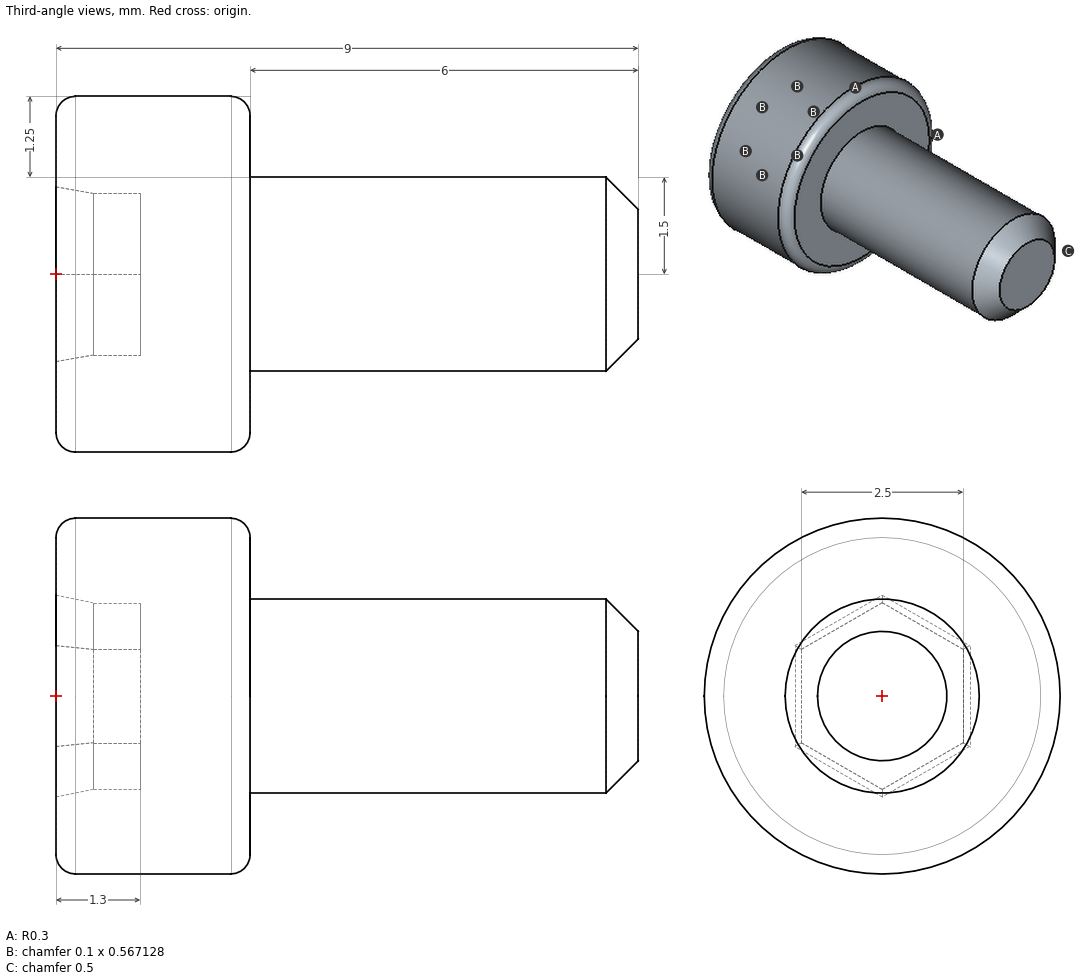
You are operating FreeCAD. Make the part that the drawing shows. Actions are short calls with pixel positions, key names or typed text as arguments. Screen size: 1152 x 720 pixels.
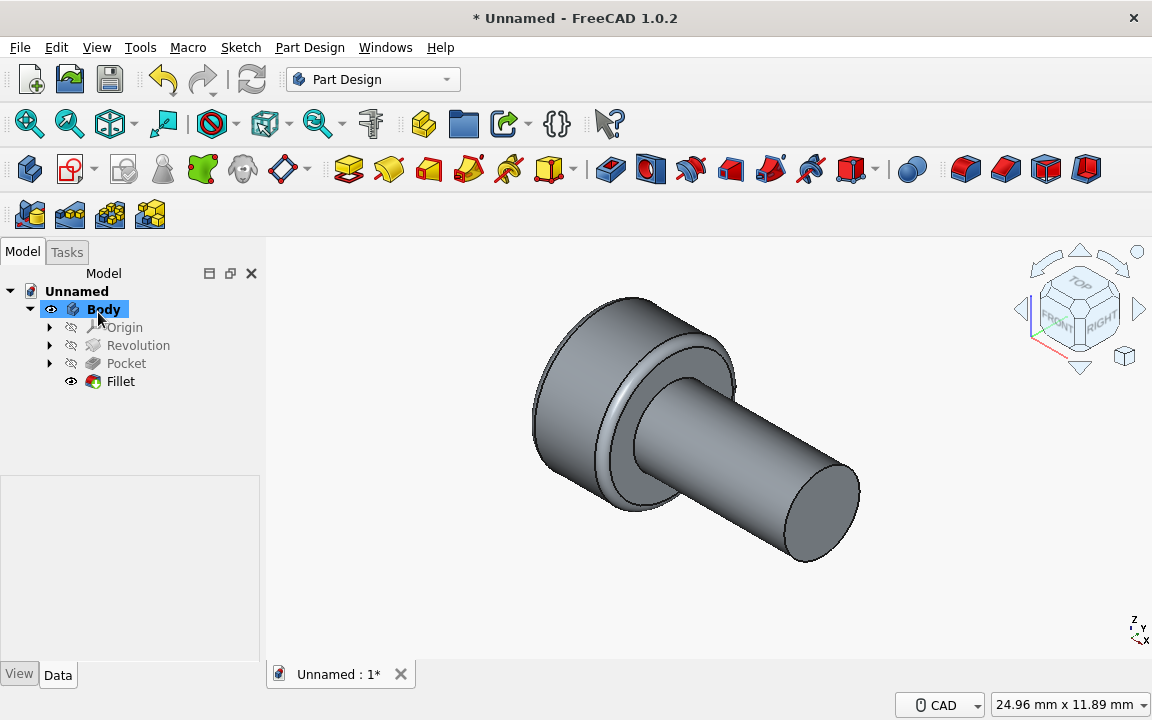
key(2)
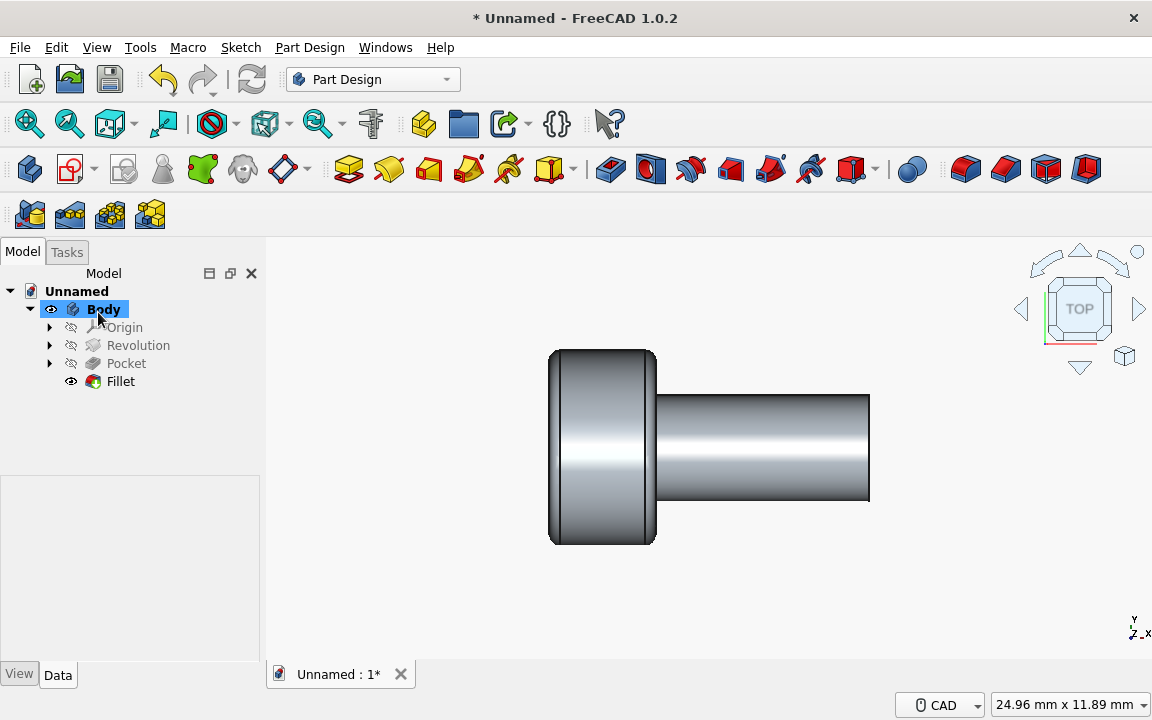
key(1)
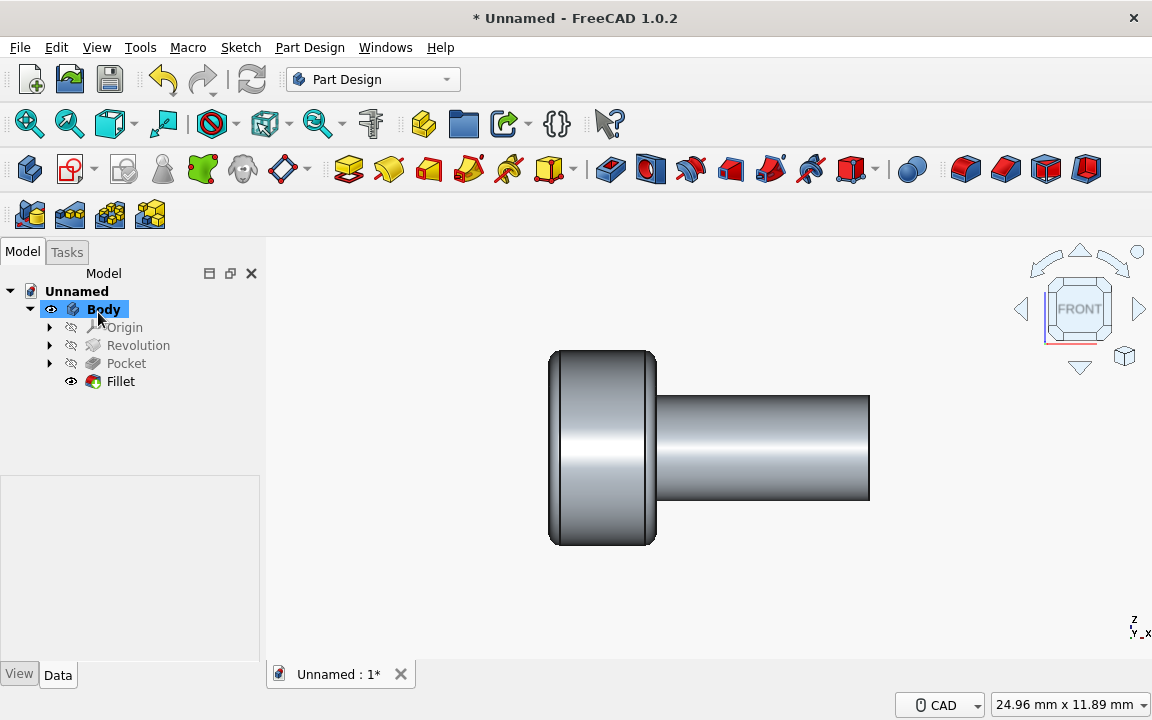
key(3)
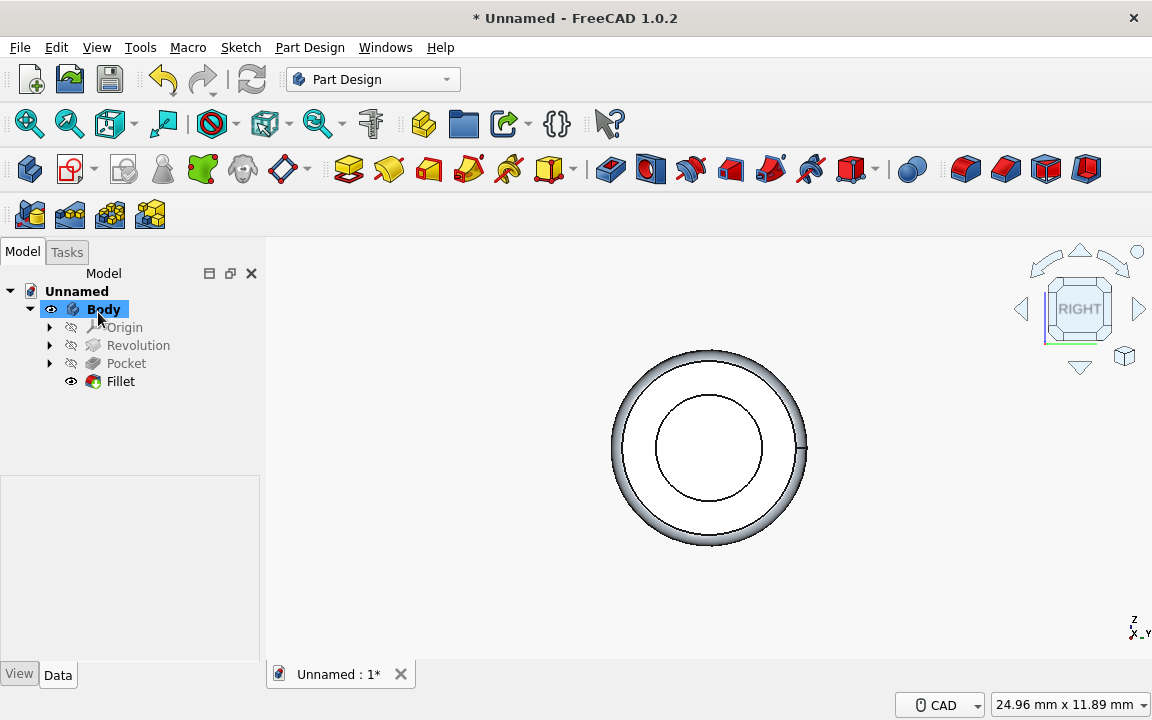
key(5)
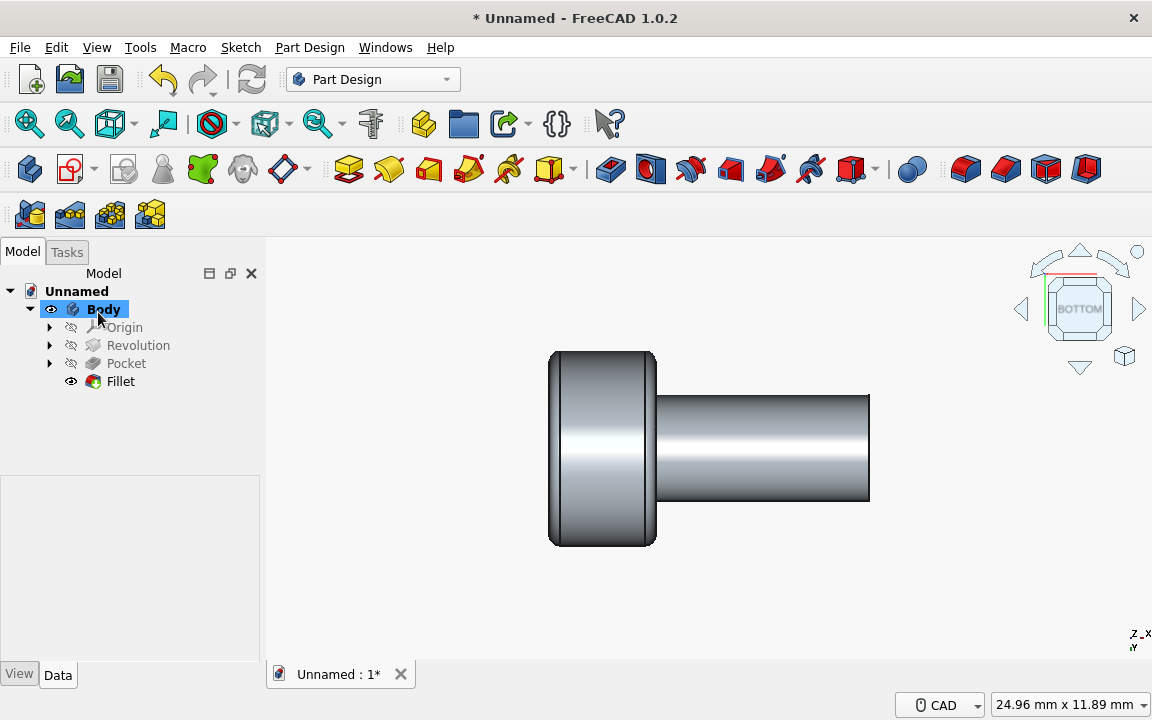
key(4)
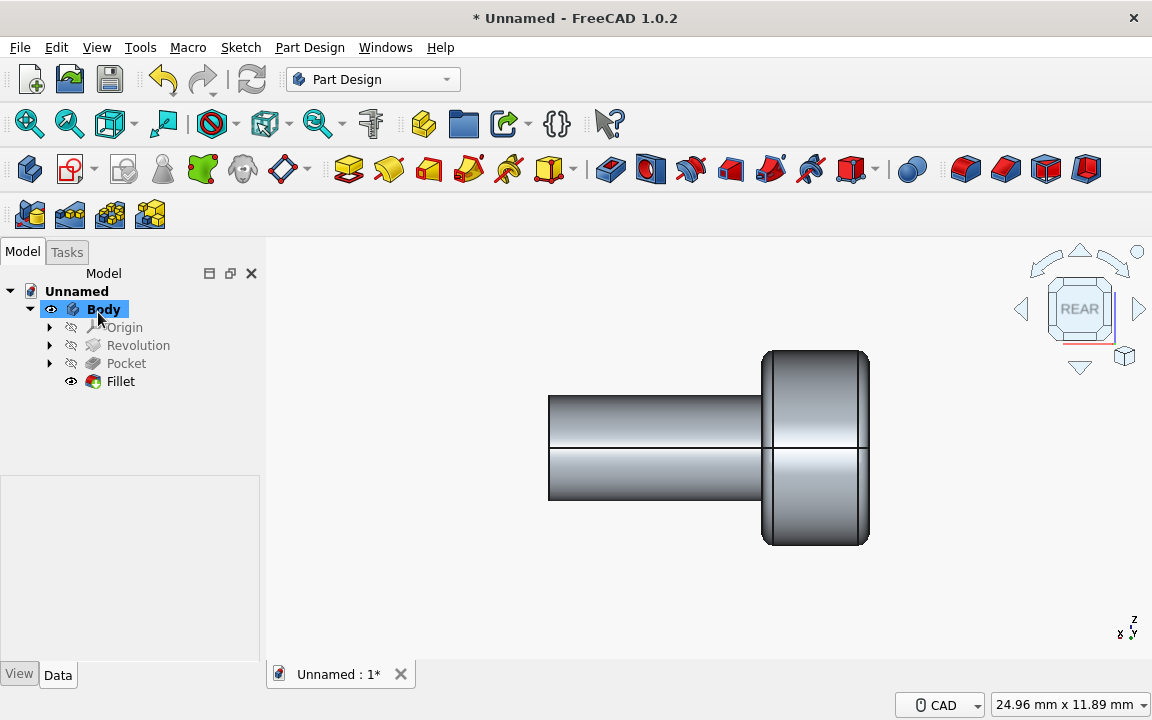
key(6)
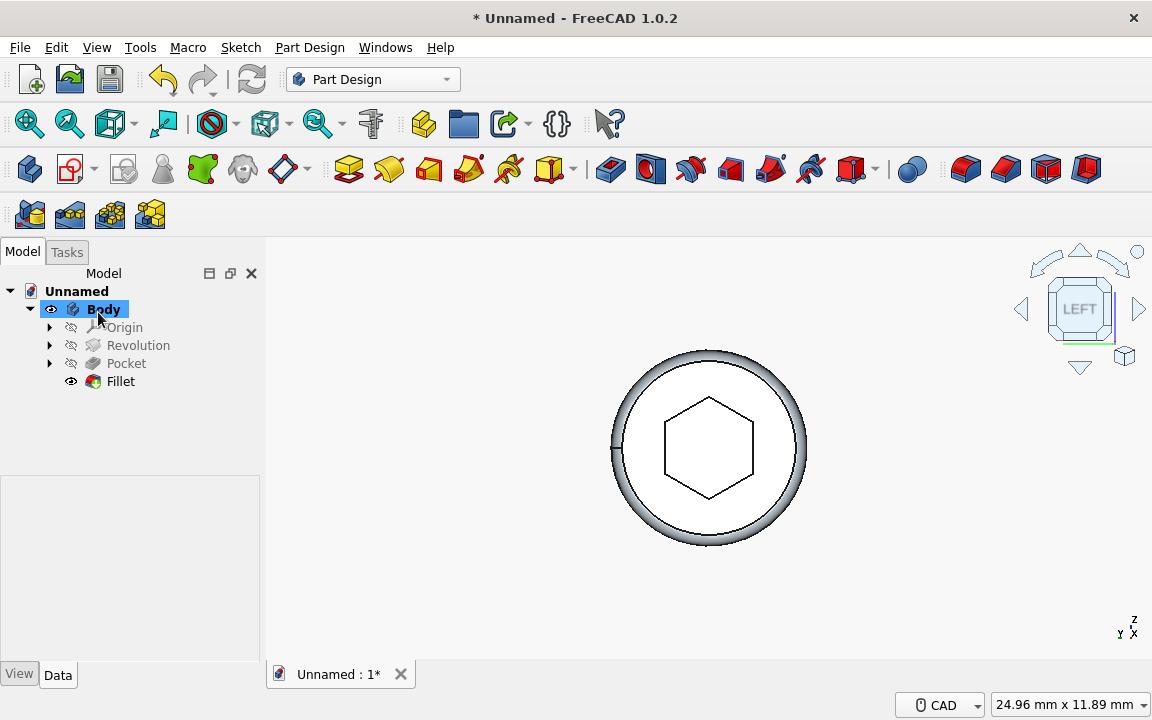
click(687, 485)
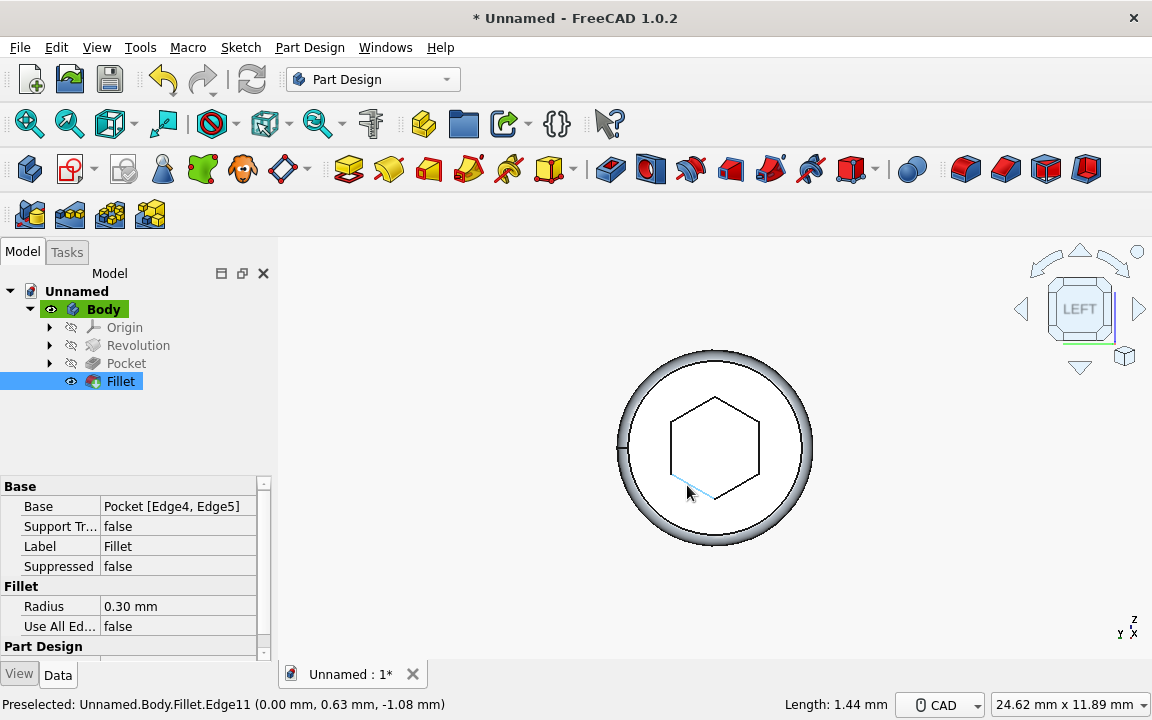
click(737, 485, ctrl)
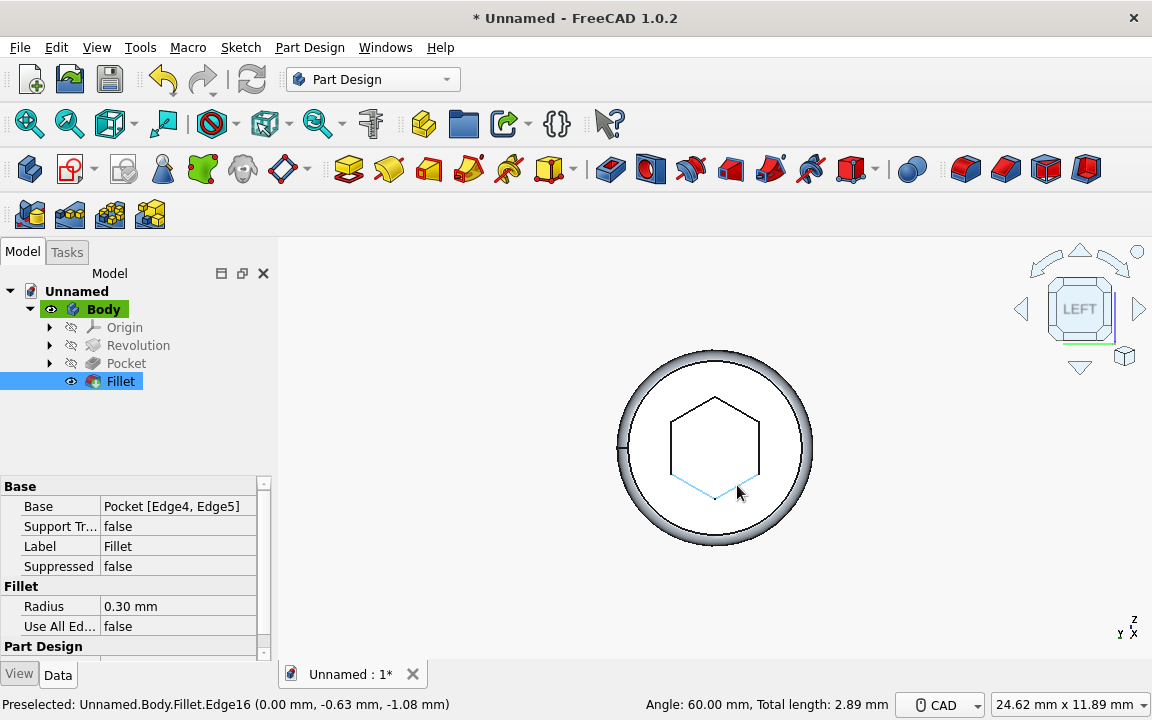
click(759, 447, ctrl)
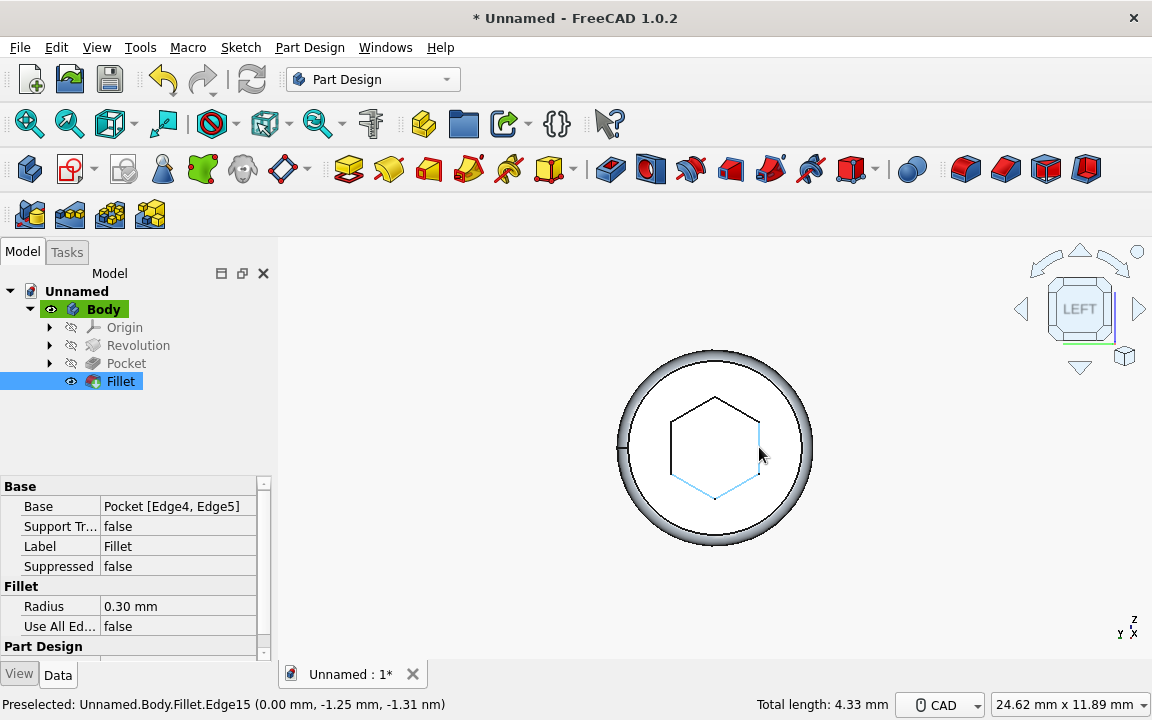
click(737, 409, ctrl)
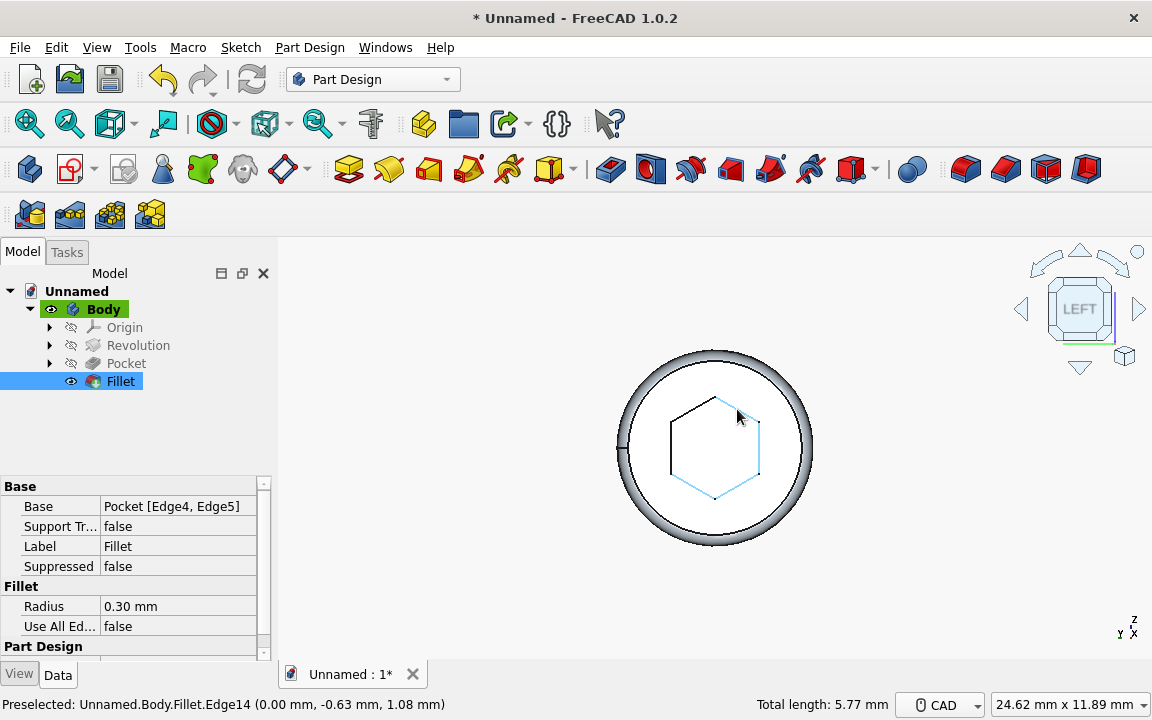
click(693, 409, ctrl)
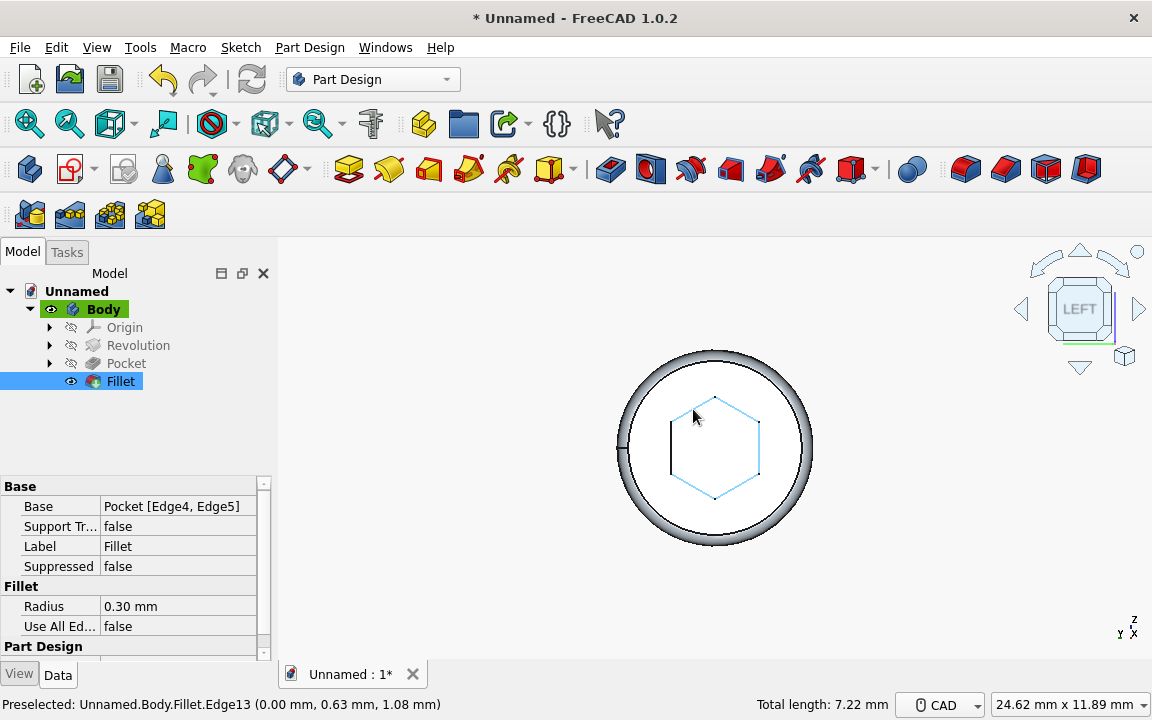
click(671, 447, ctrl)